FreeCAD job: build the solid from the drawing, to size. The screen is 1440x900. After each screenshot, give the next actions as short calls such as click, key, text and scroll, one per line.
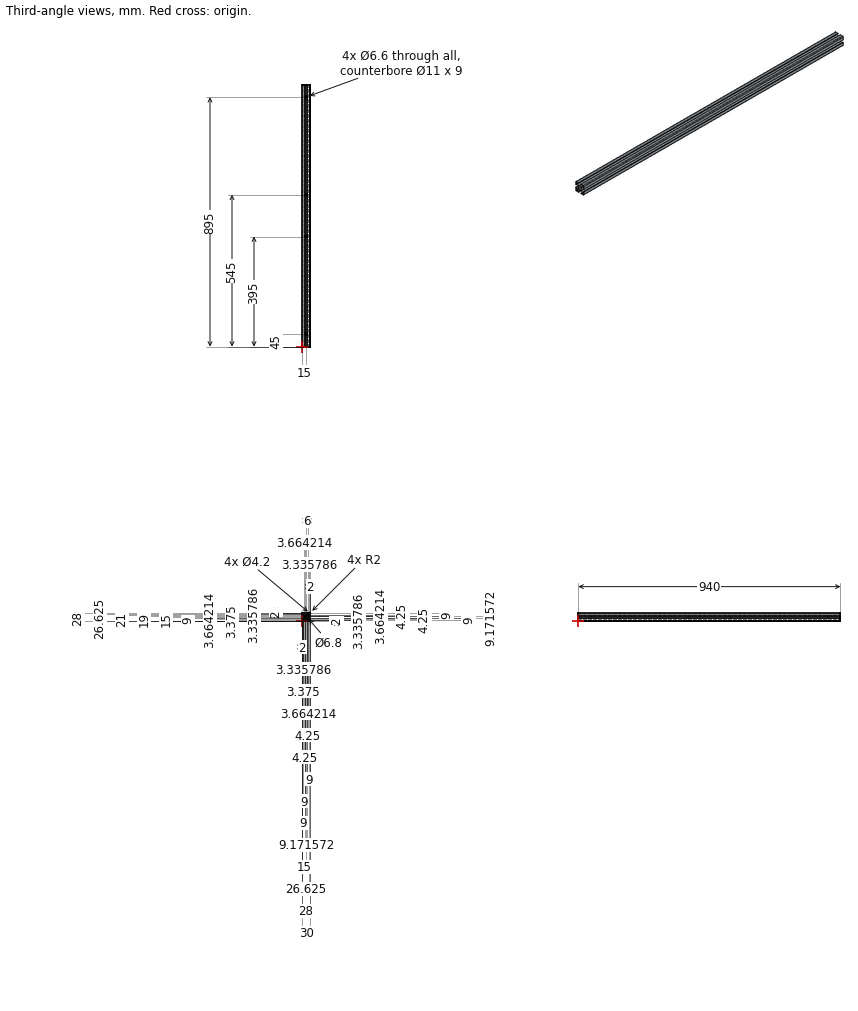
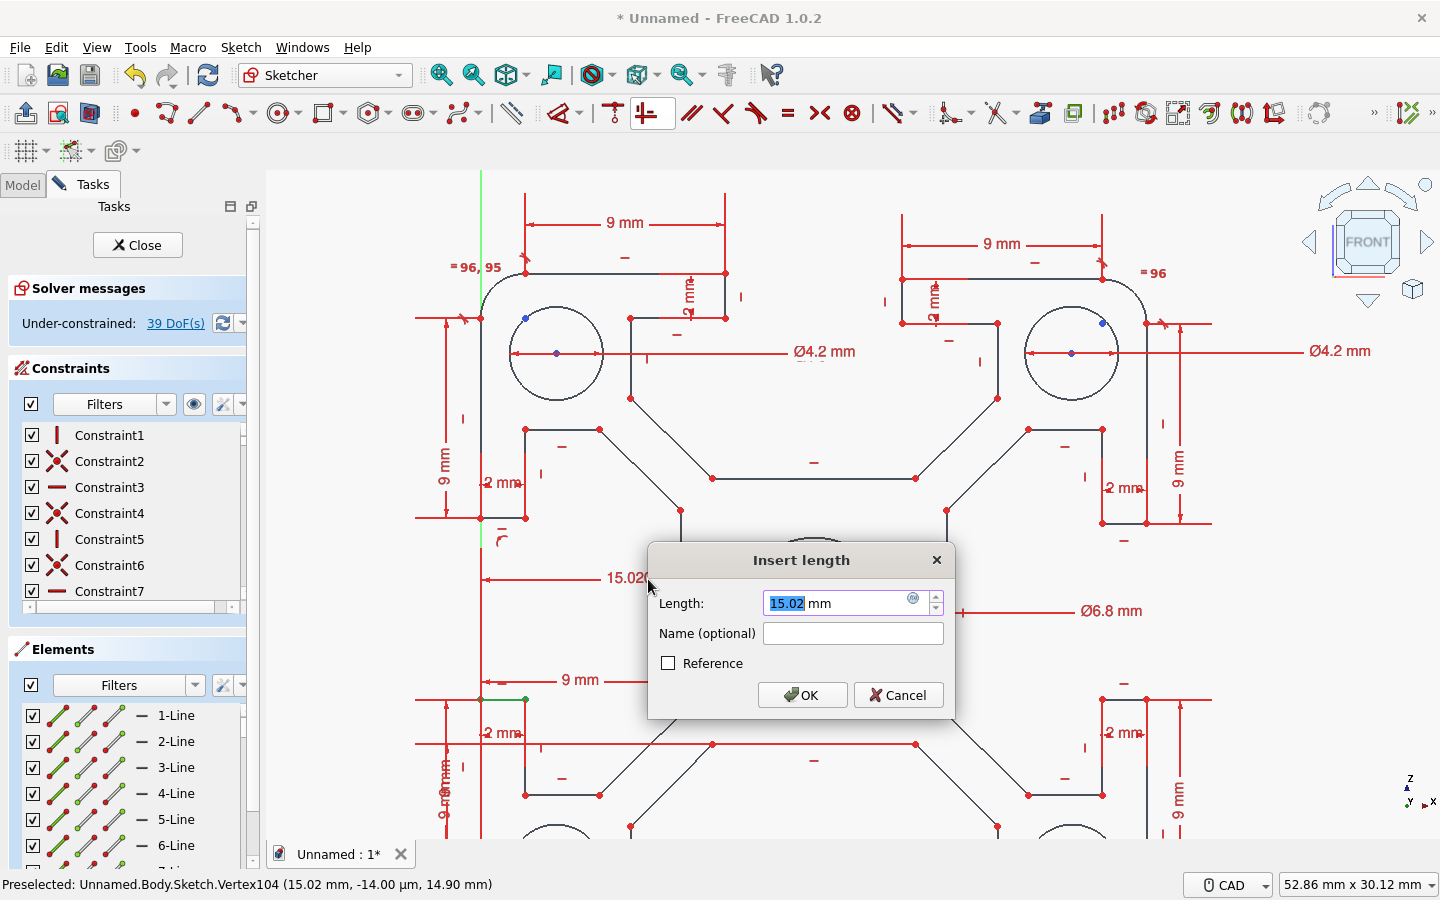
text(15)
key(Return)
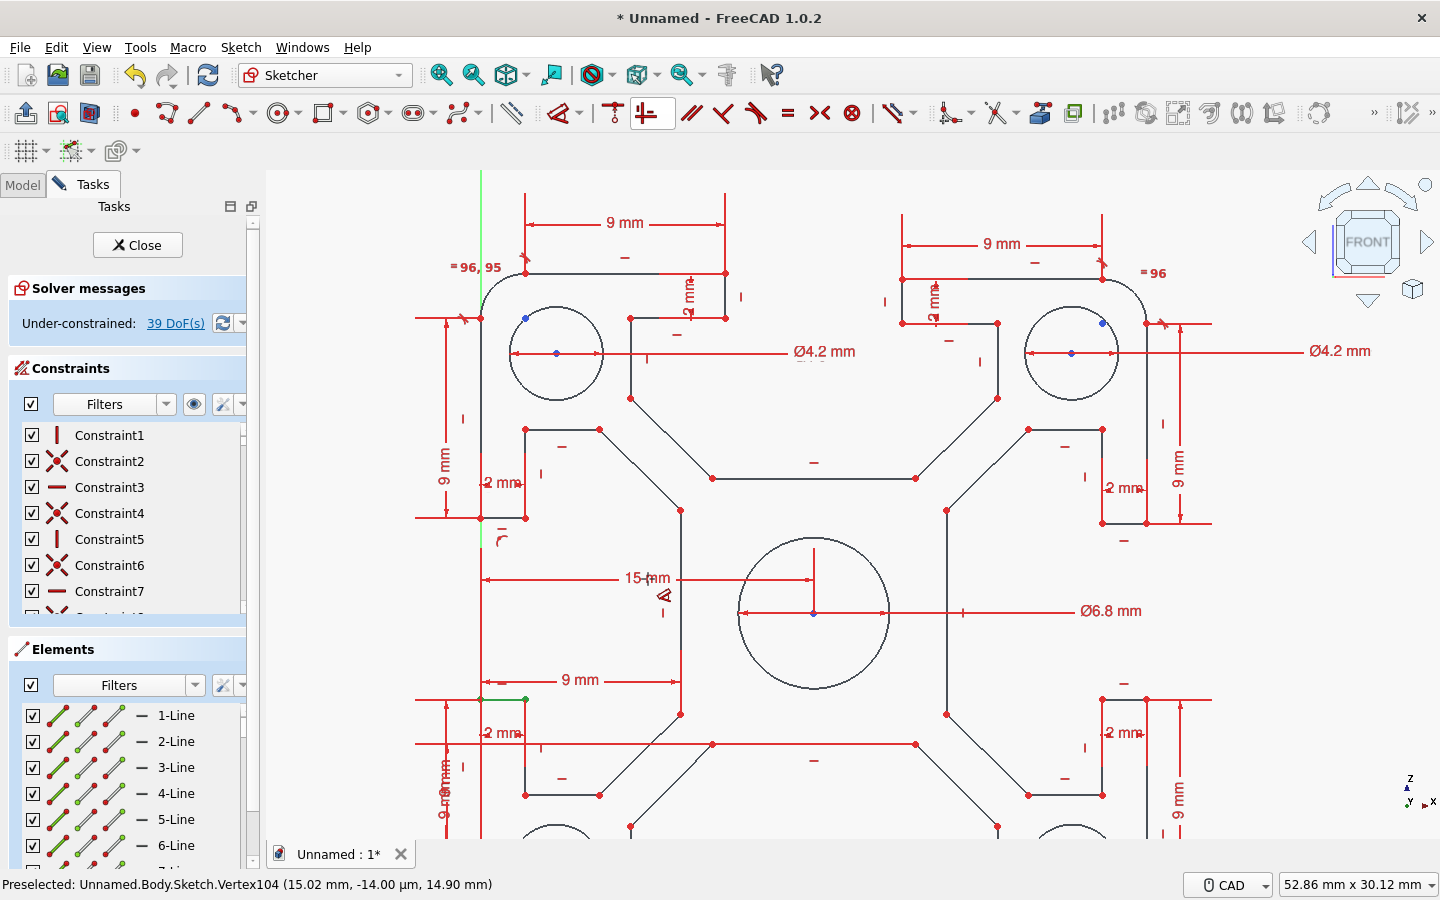
click(814, 613)
click(447, 712)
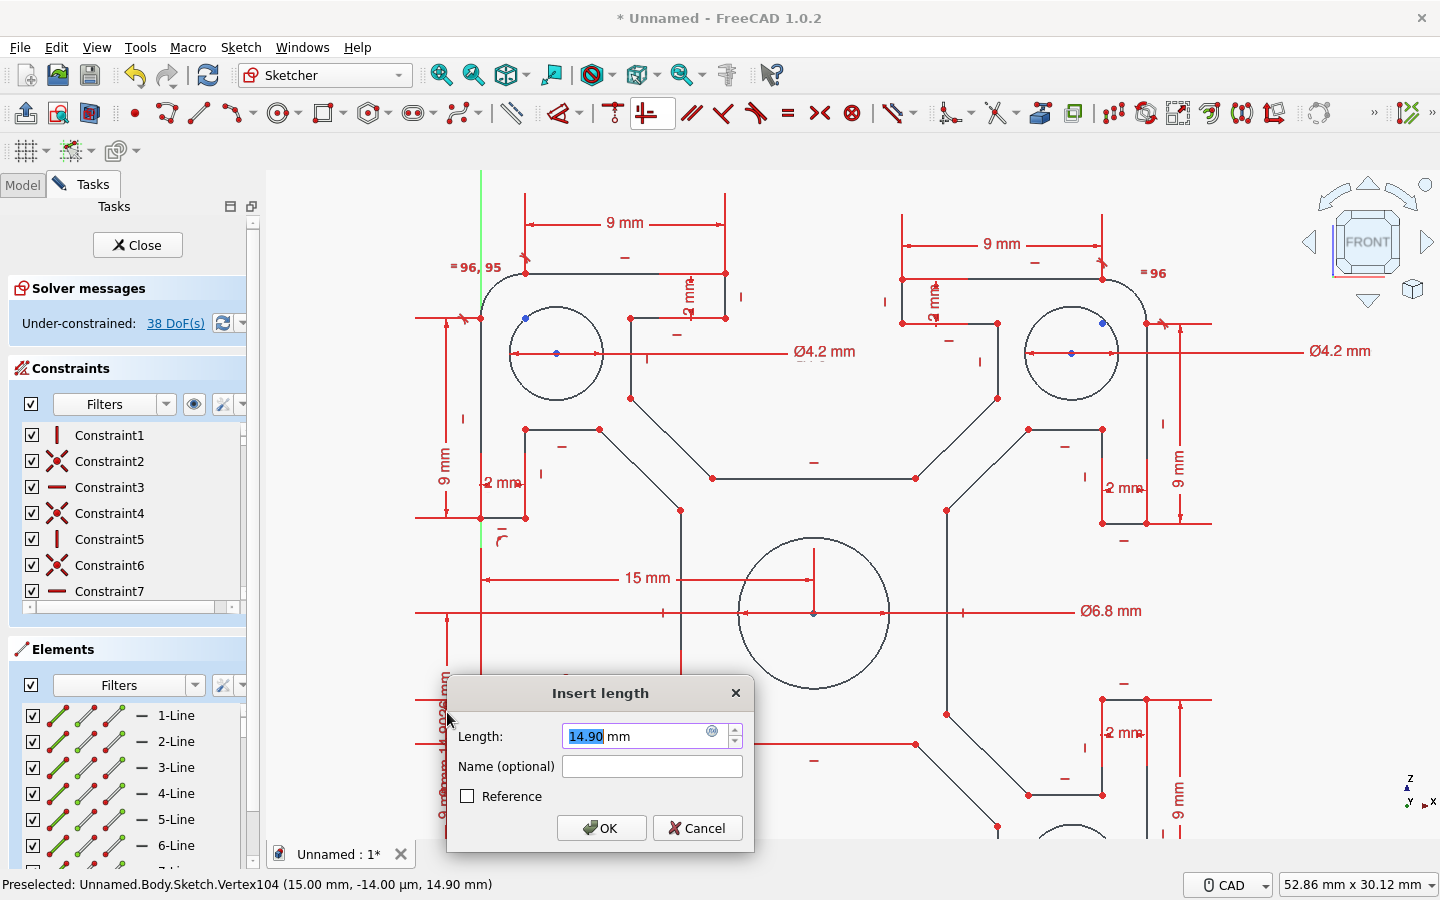
text(15)
key(Return)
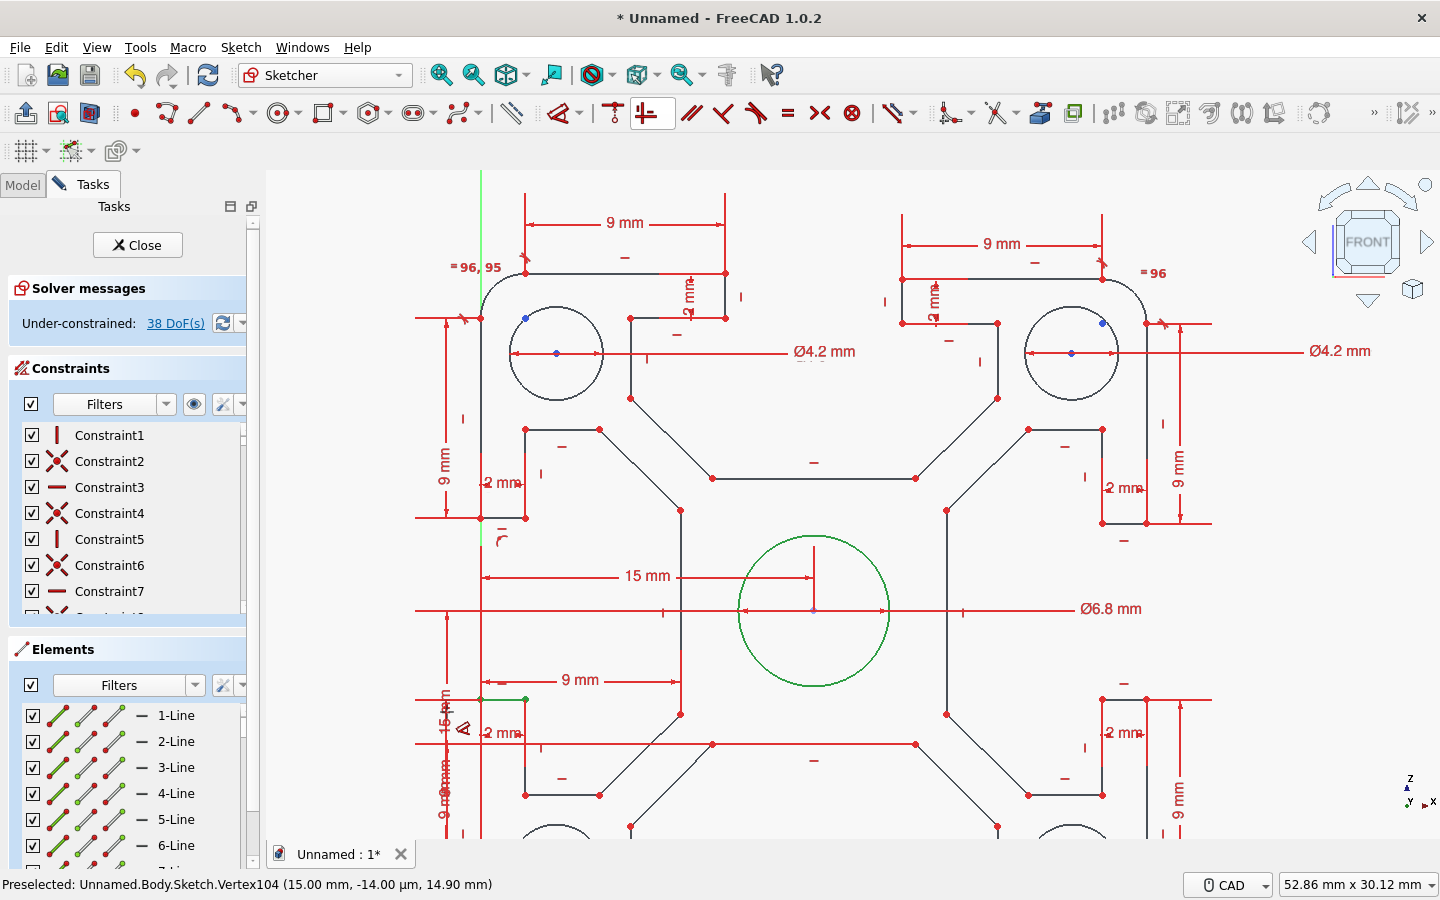
click(947, 510)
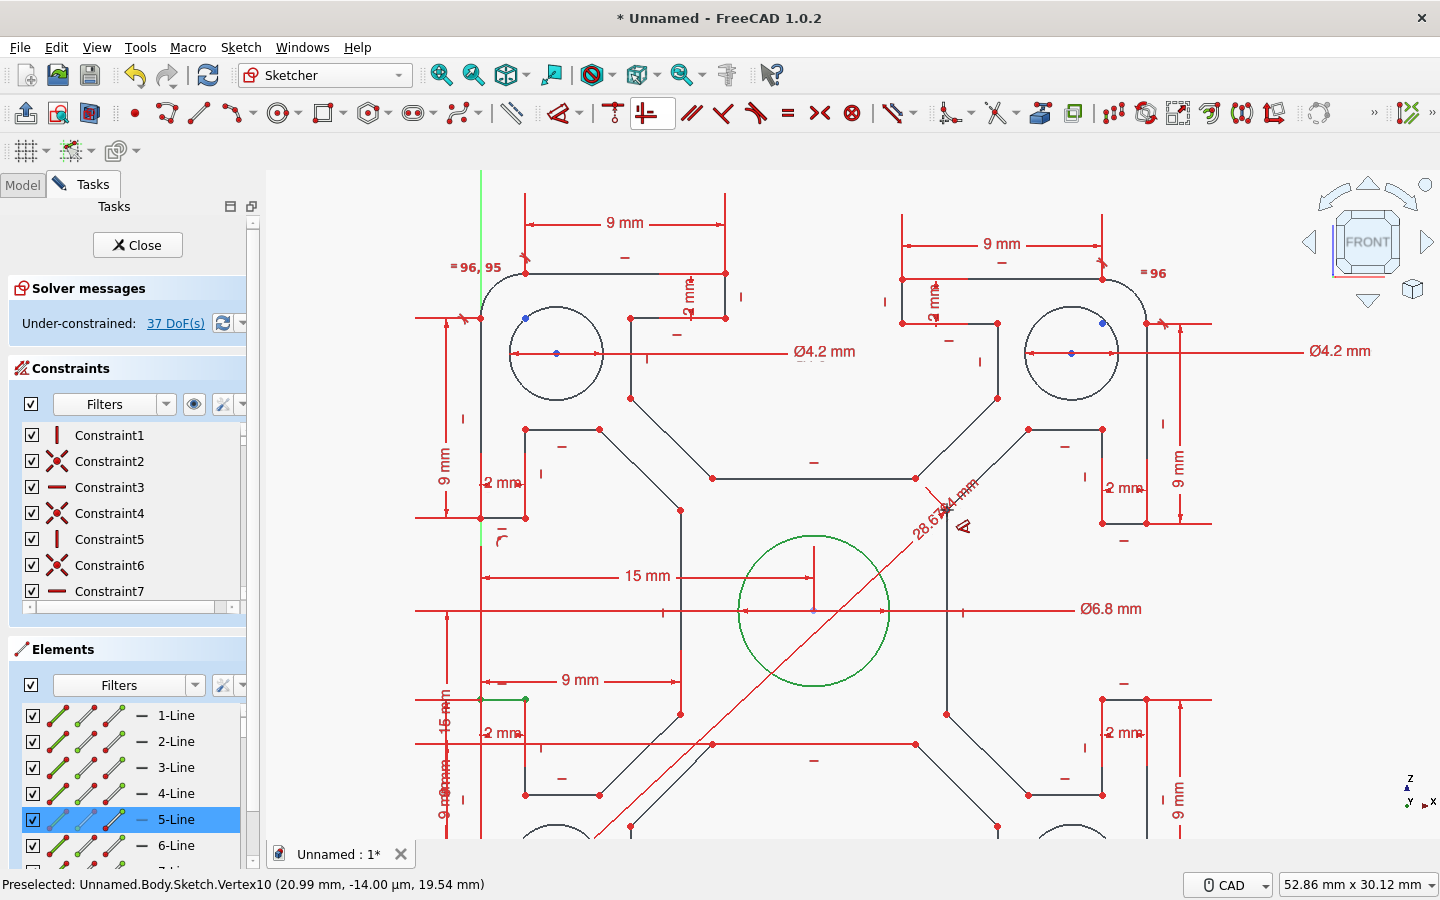
click(814, 611)
click(850, 645)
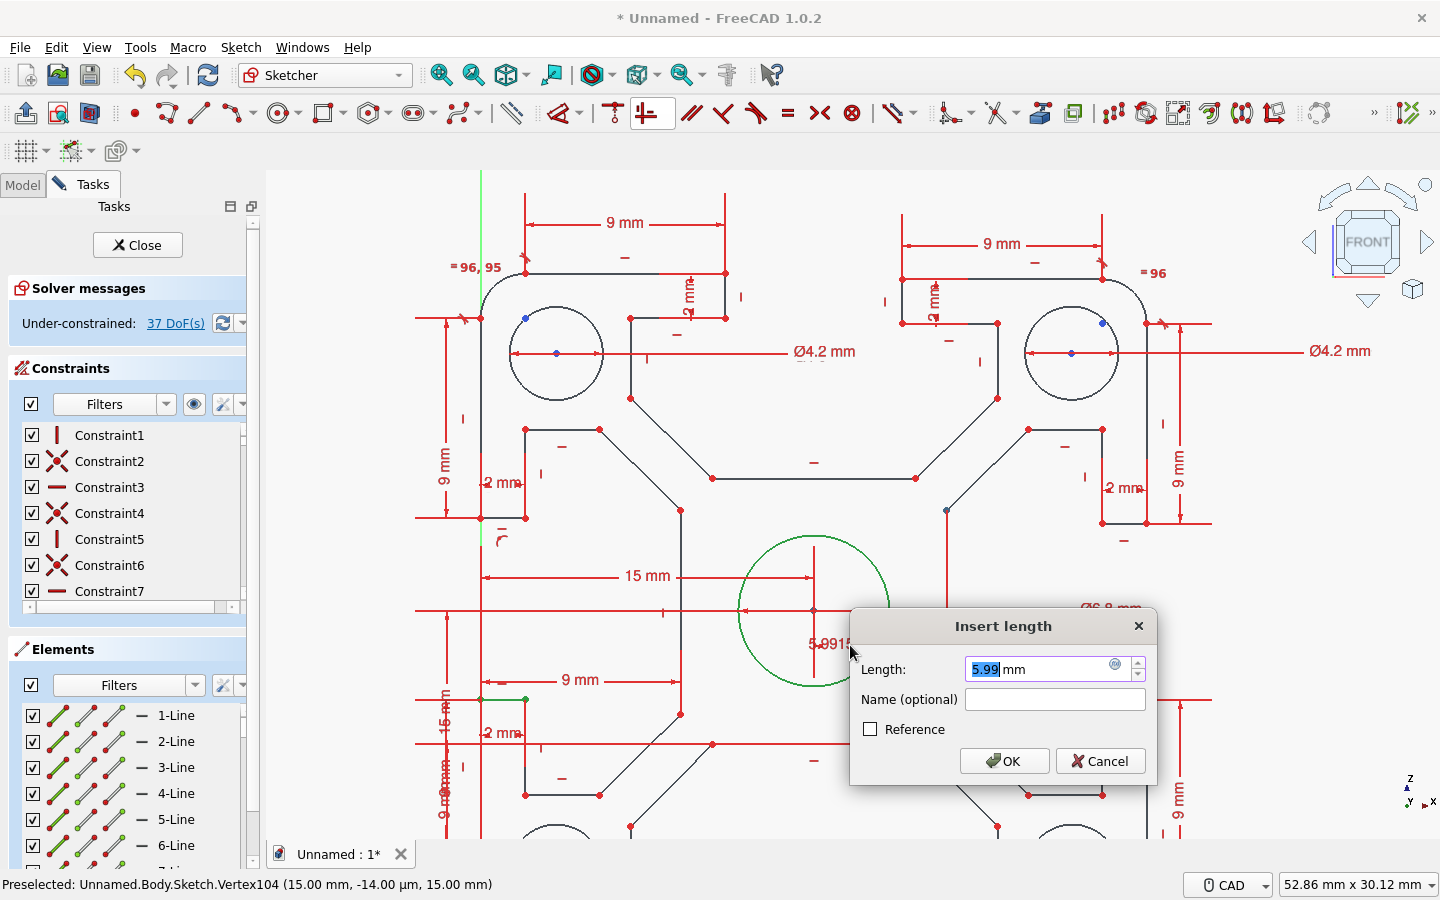
text(6)
key(Return)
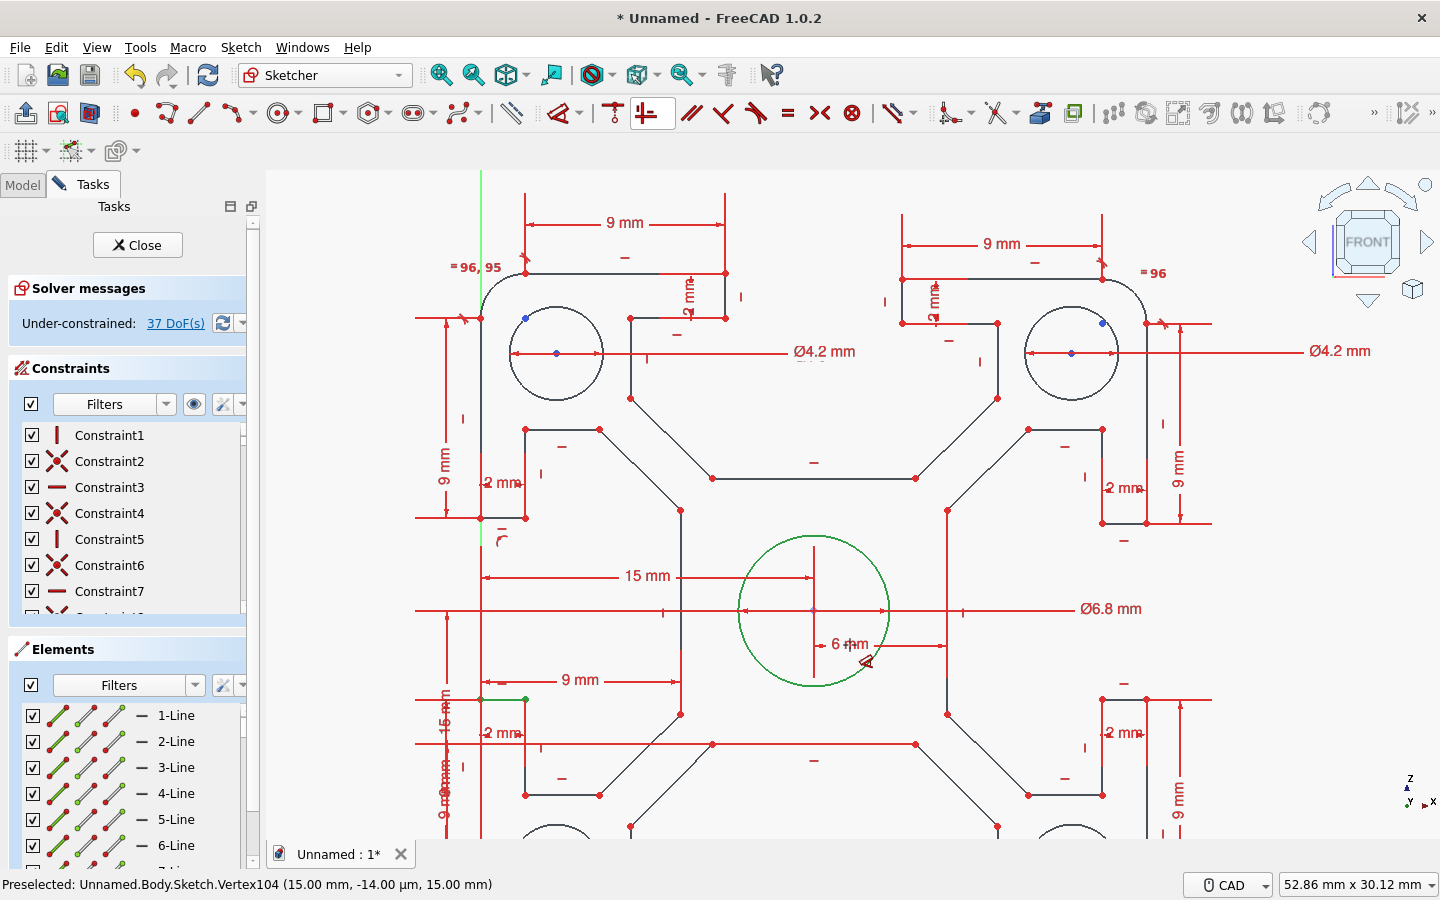
click(1147, 324)
click(814, 290)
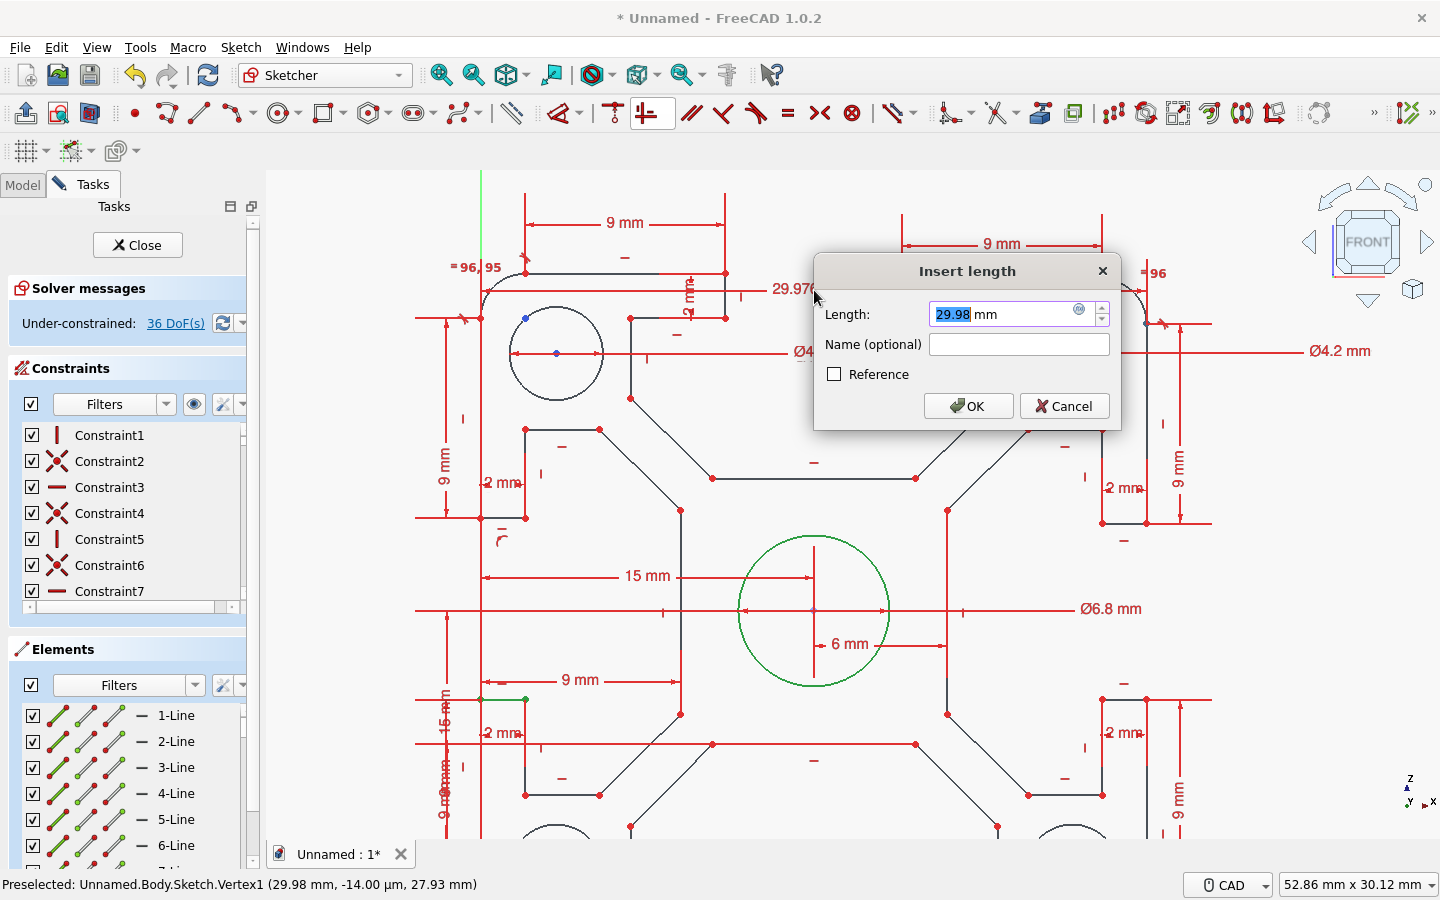
text(30)
key(Return)